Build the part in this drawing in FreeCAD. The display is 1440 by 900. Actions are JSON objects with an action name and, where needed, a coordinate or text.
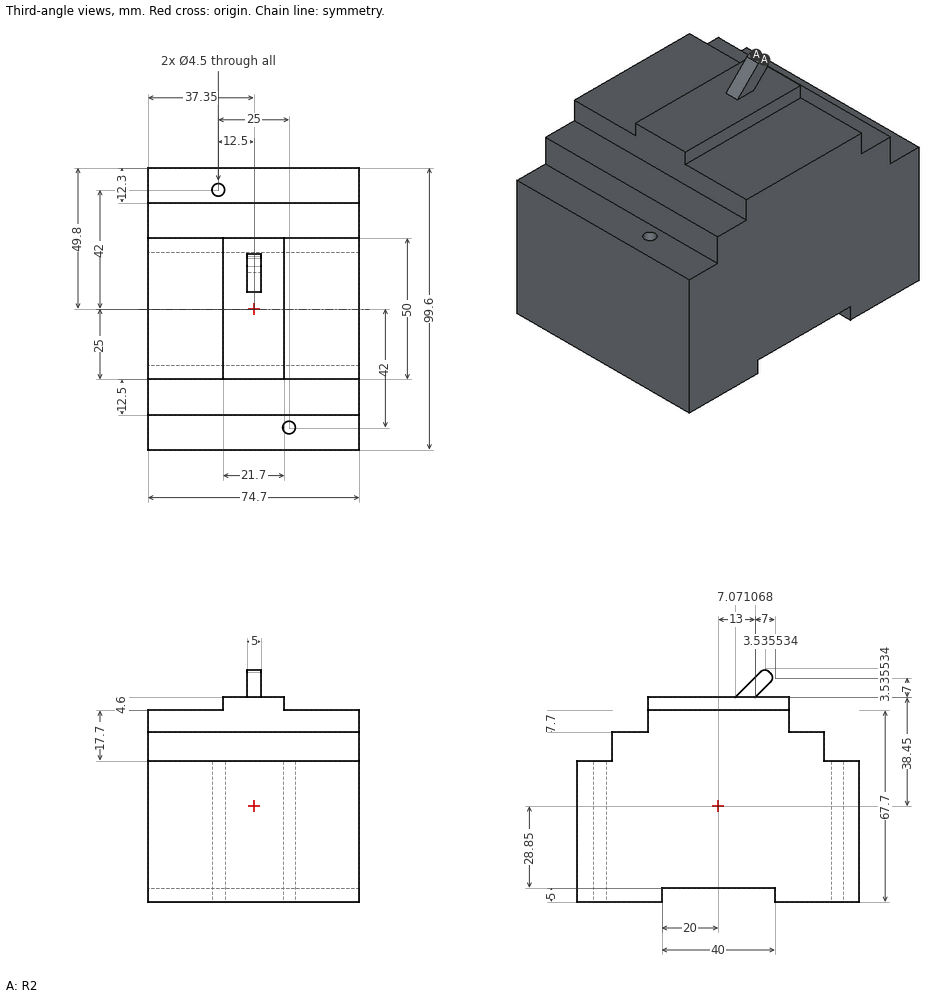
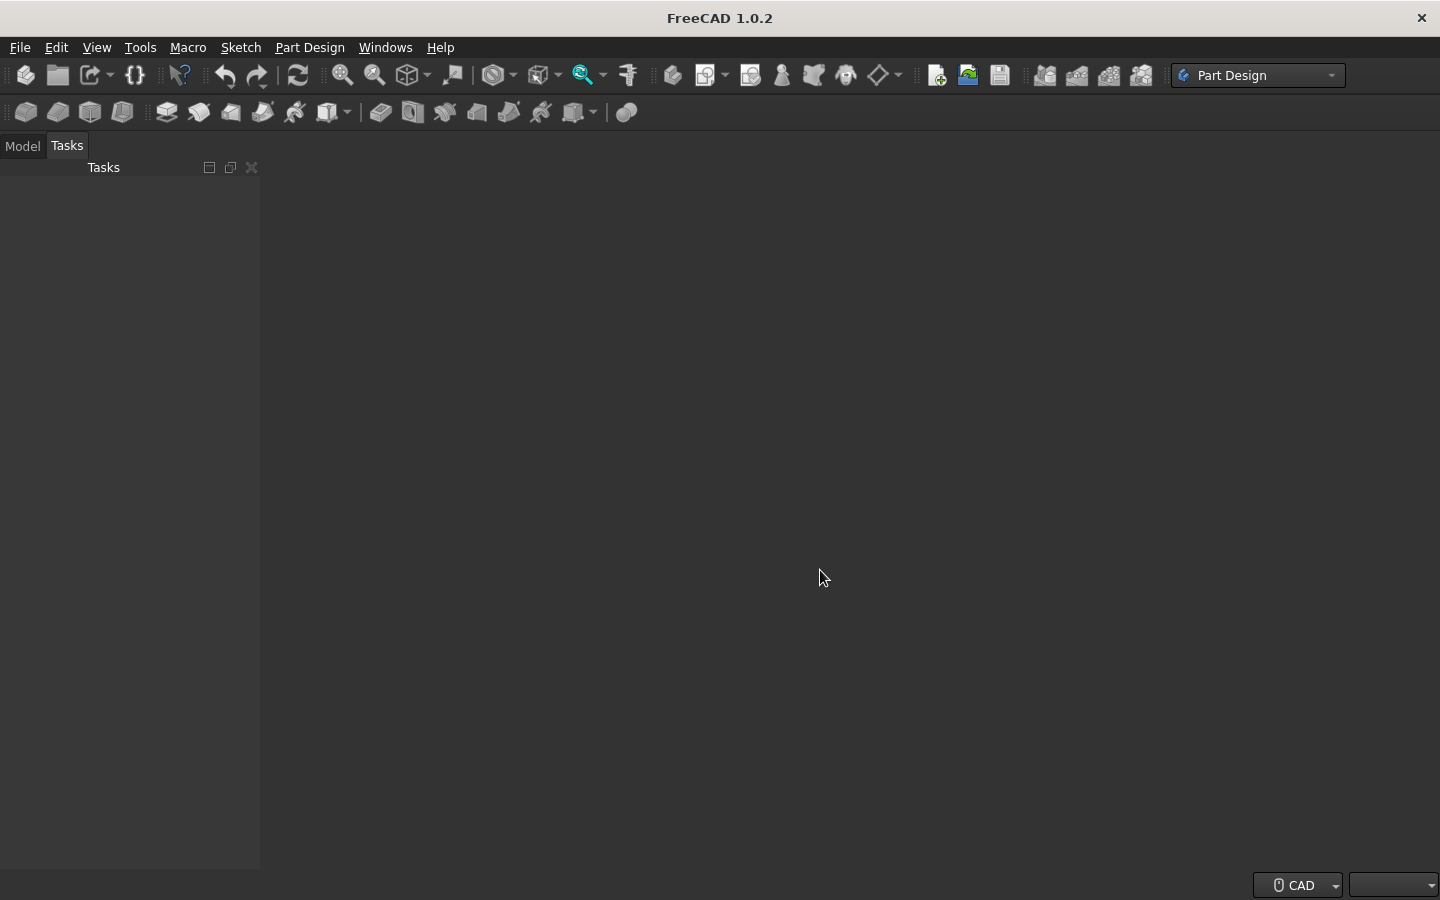
{"action": "left_click", "coordinate": [936, 76]}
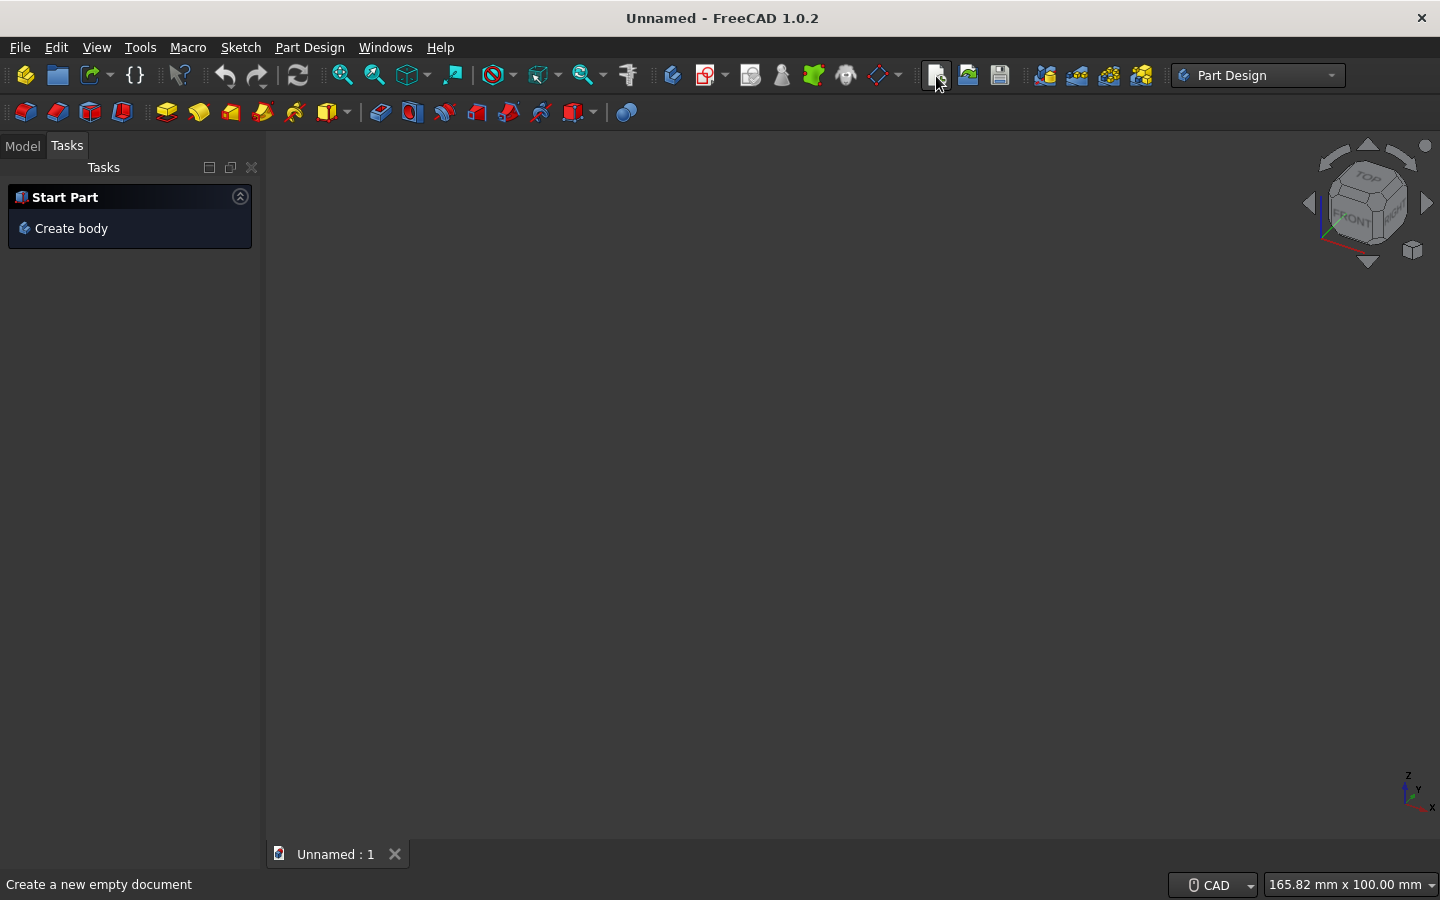
{"action": "left_click", "coordinate": [706, 76]}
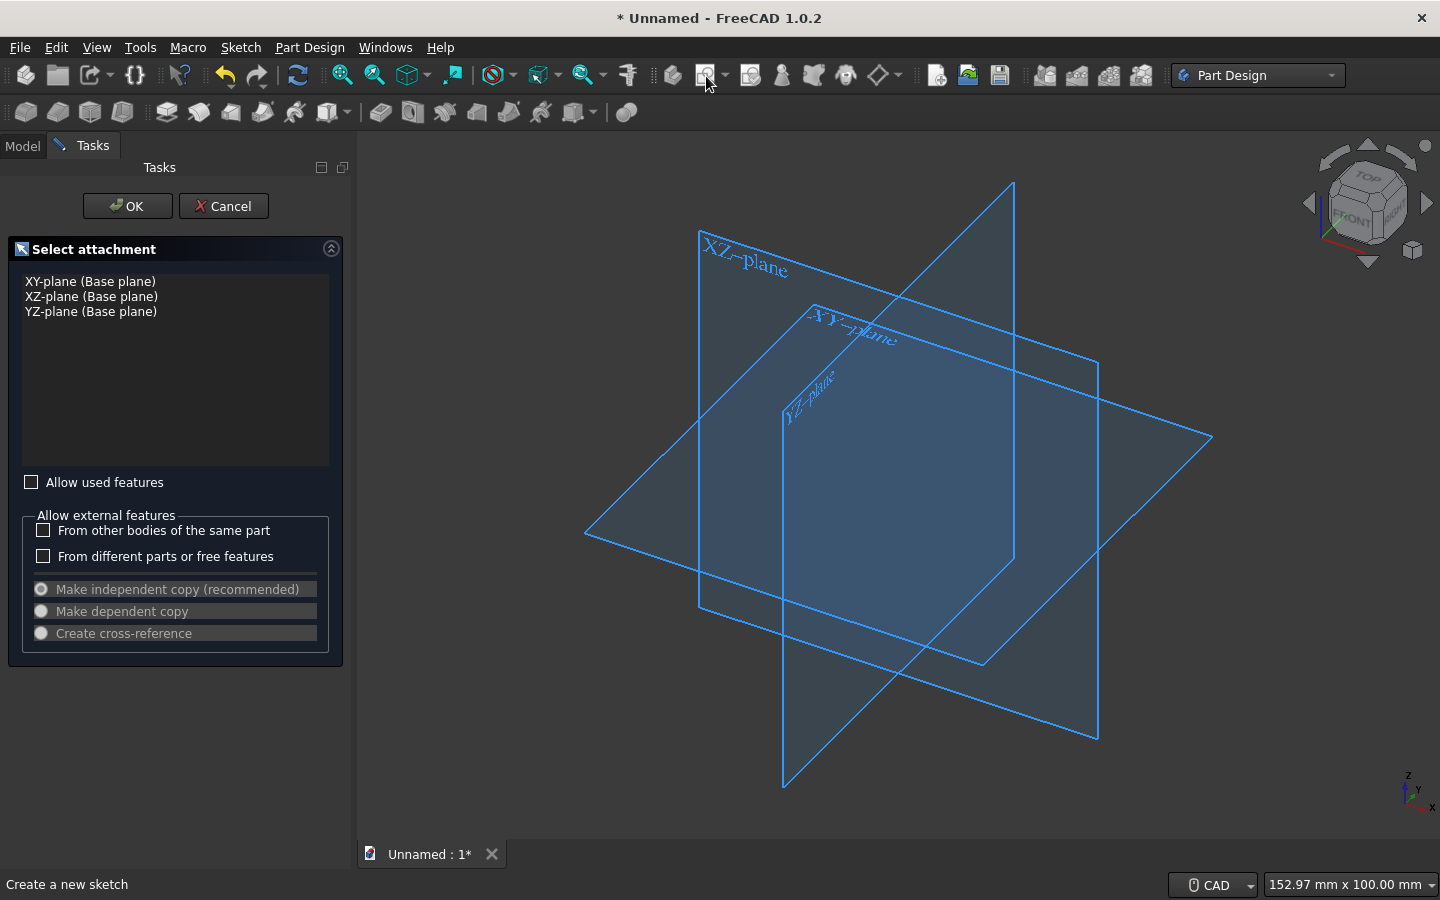
{"action": "left_click", "coordinate": [82, 282]}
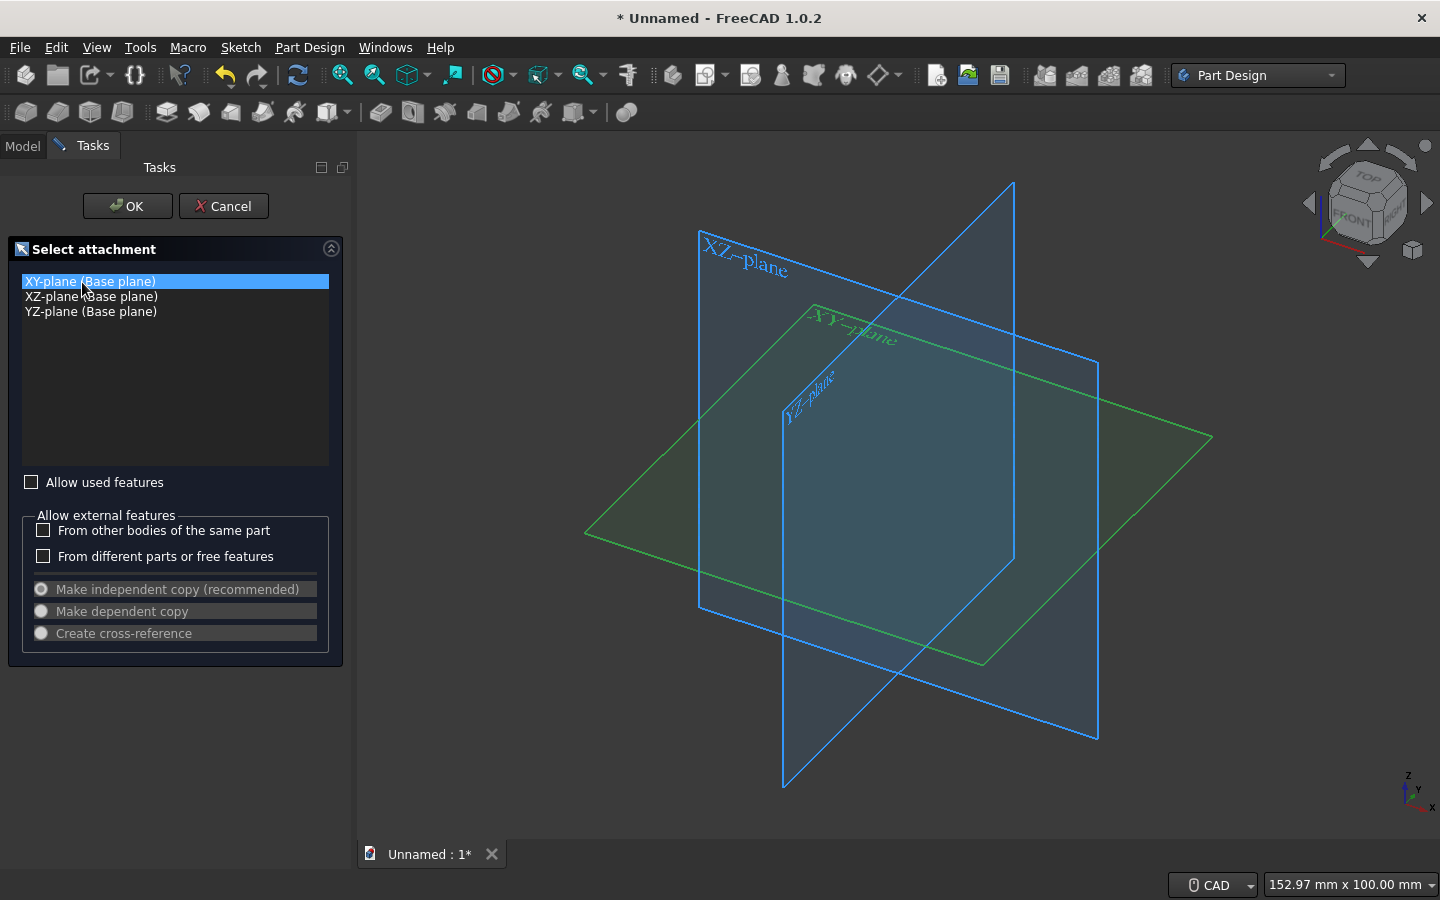
{"action": "left_click", "coordinate": [128, 206]}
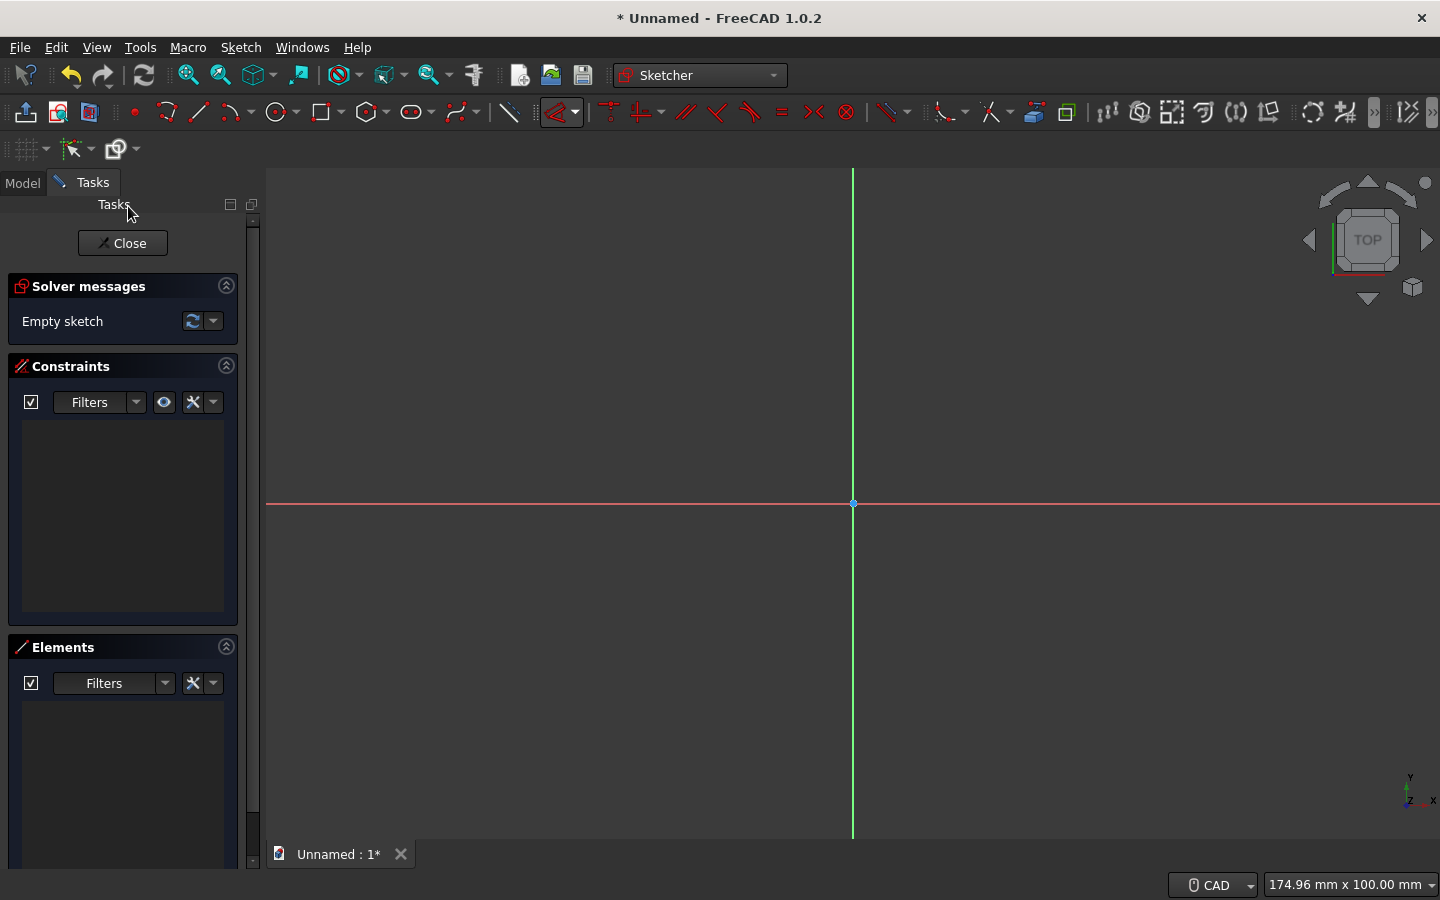
{"action": "scroll", "coordinate": [645, 504], "scroll_direction": "down", "scroll_amount": 2}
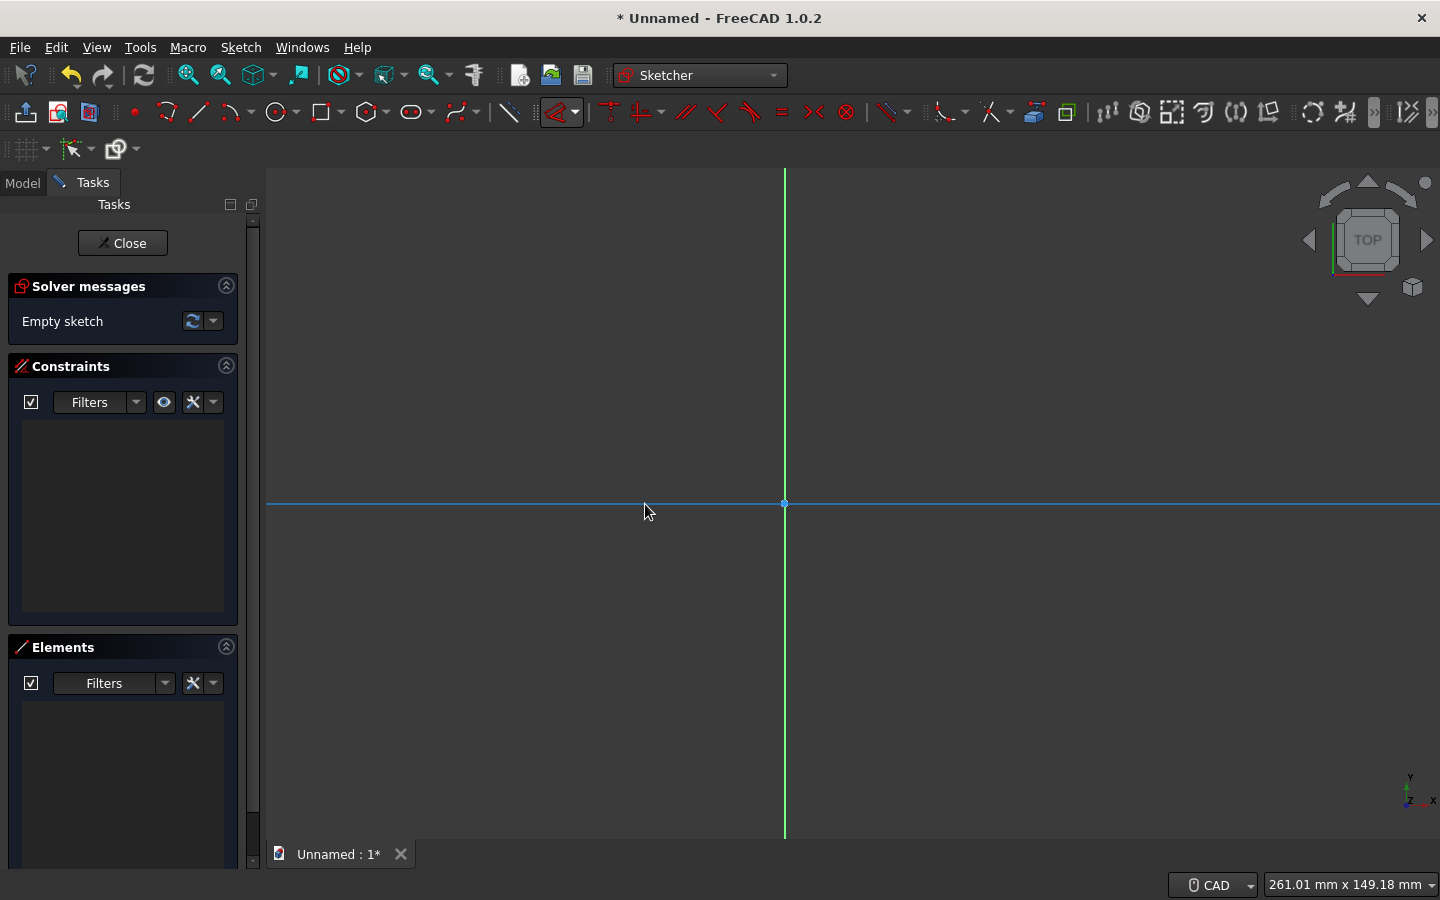
{"action": "left_click", "coordinate": [344, 112]}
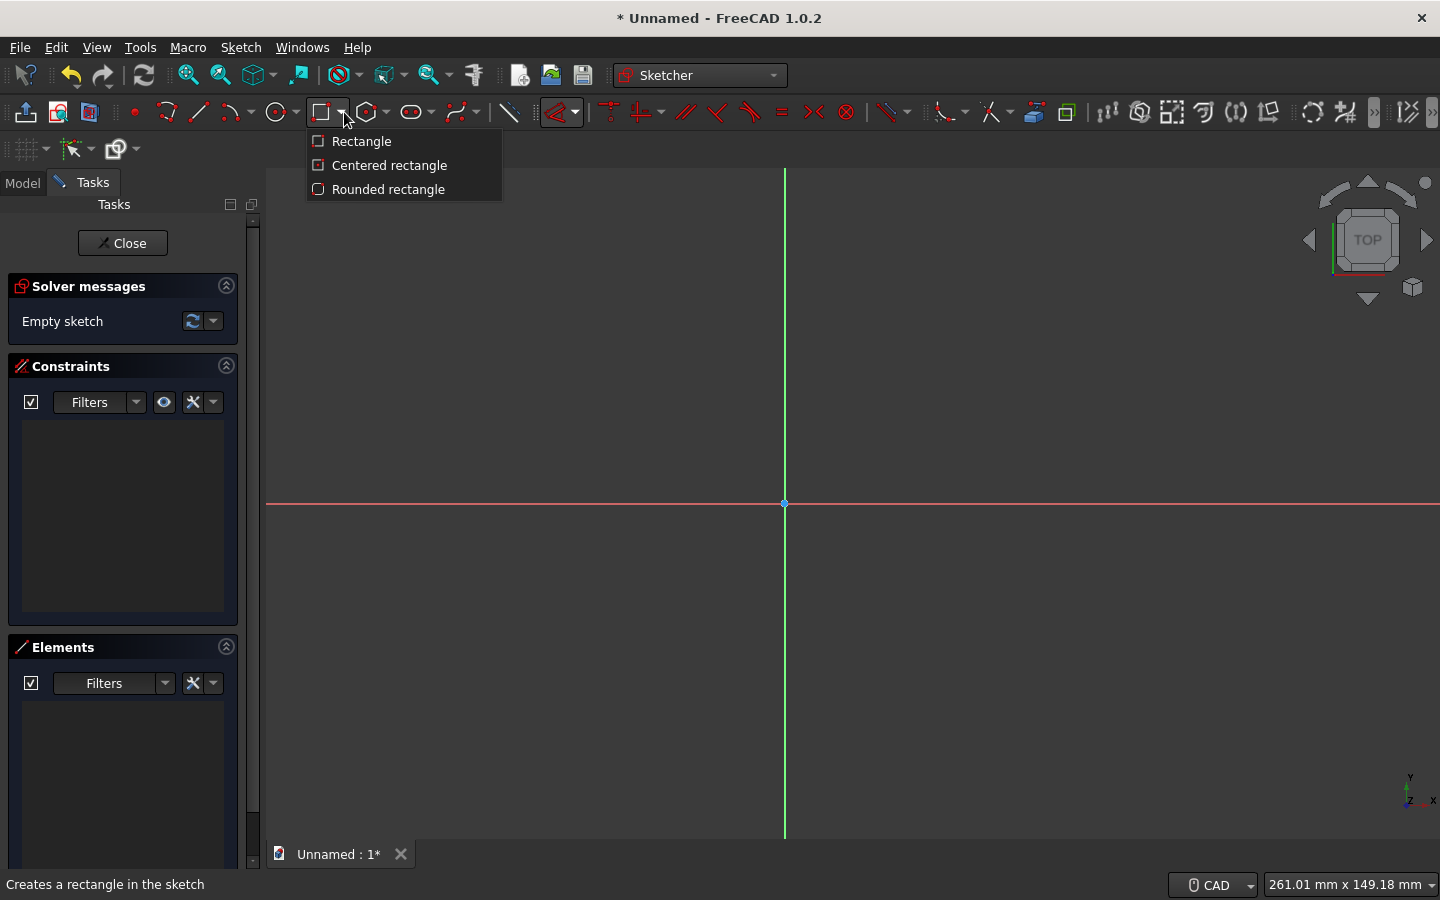
{"action": "left_click", "coordinate": [404, 165]}